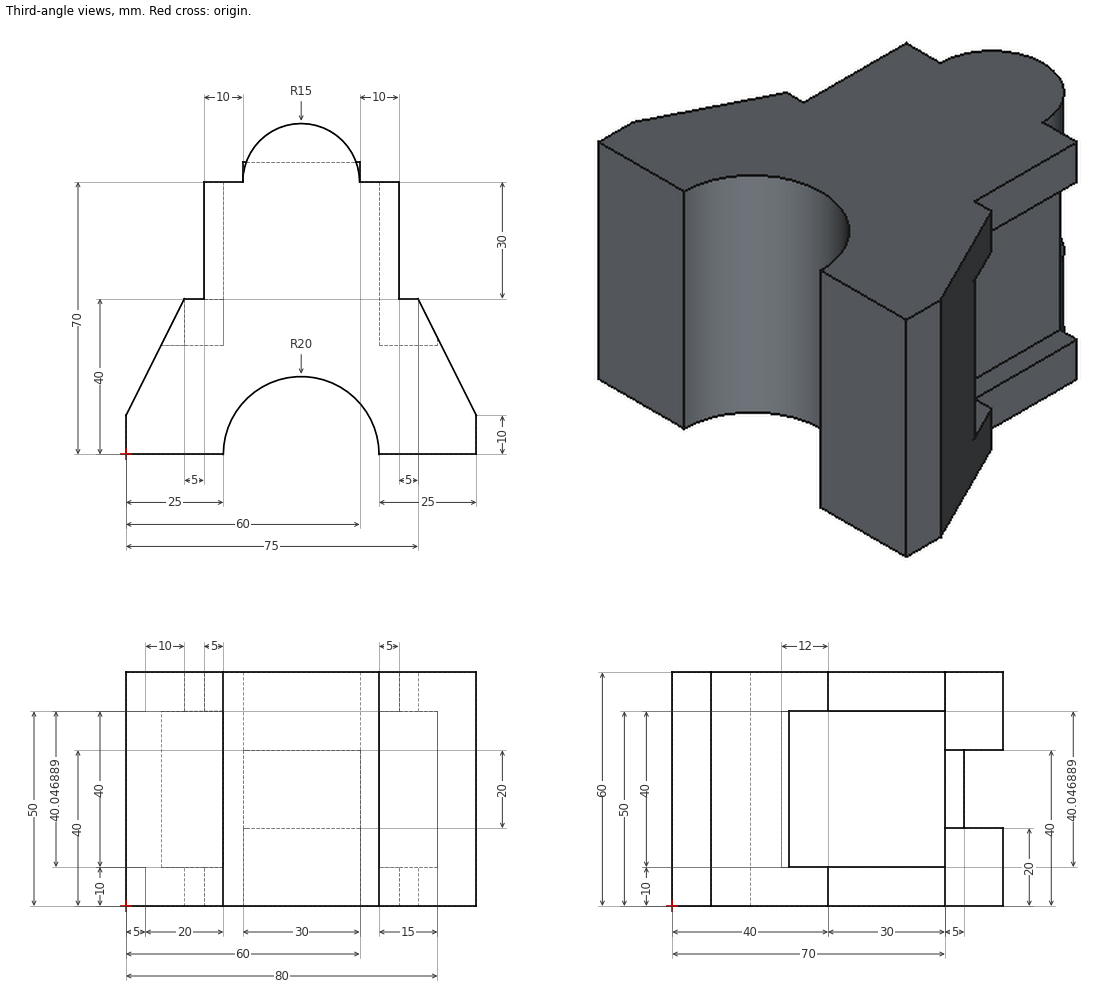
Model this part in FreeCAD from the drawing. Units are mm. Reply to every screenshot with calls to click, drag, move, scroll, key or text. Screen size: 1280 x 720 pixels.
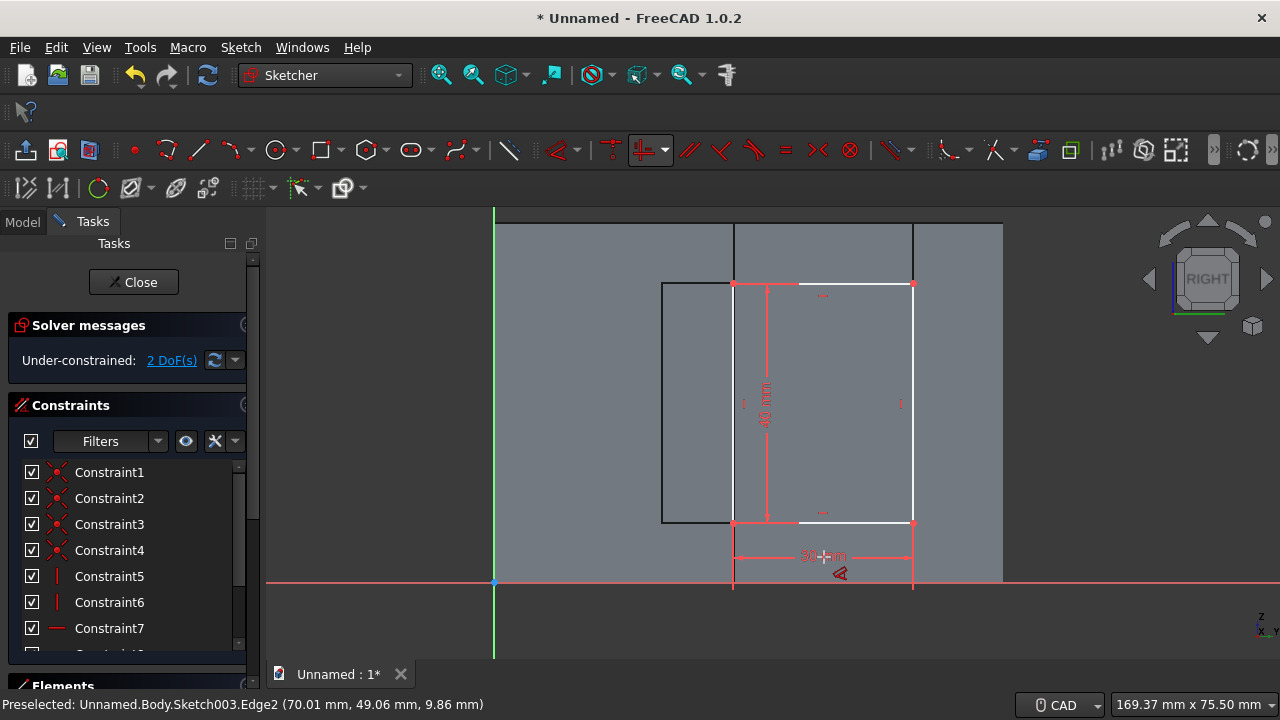
click(733, 284)
click(614, 617)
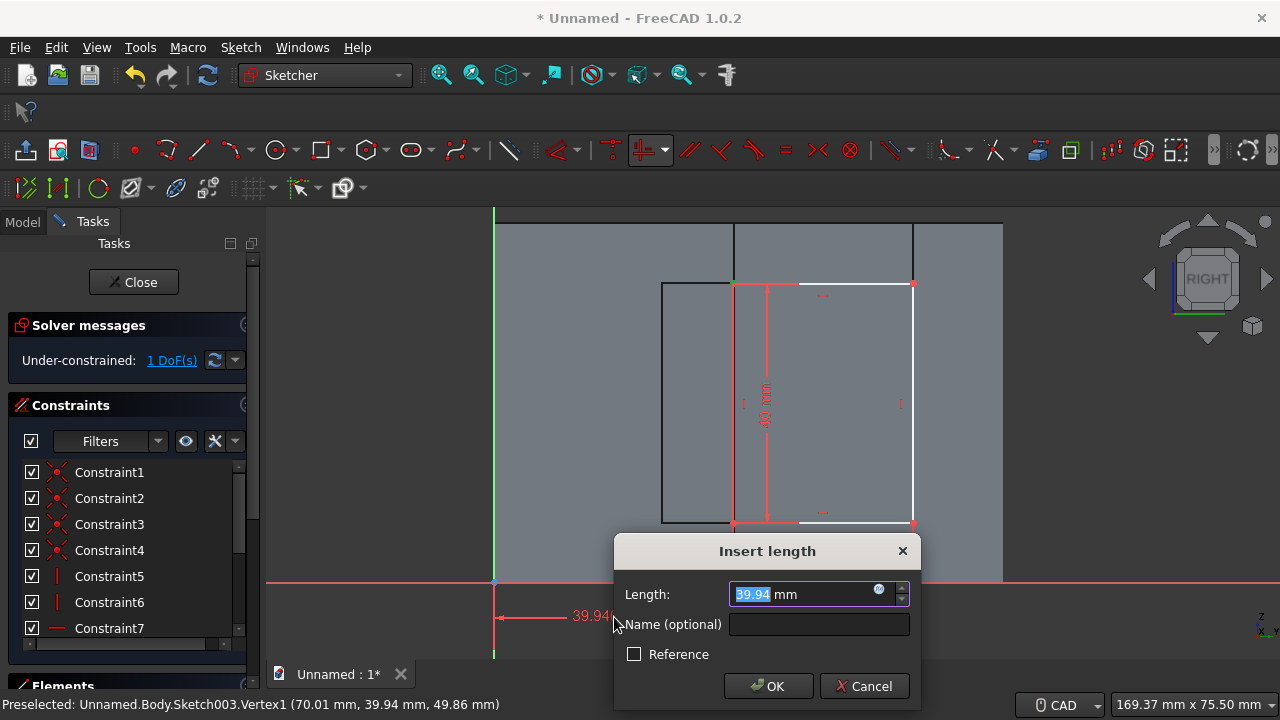
text(40)
key(Return)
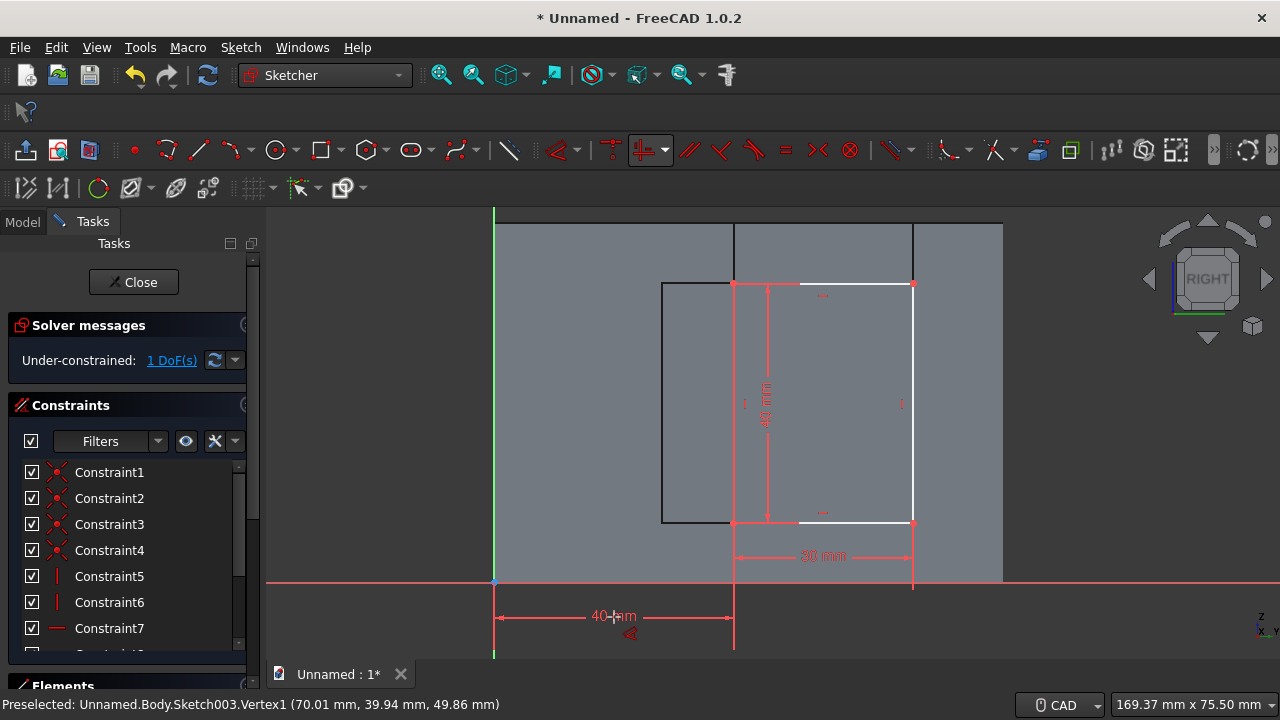
click(734, 284)
click(460, 433)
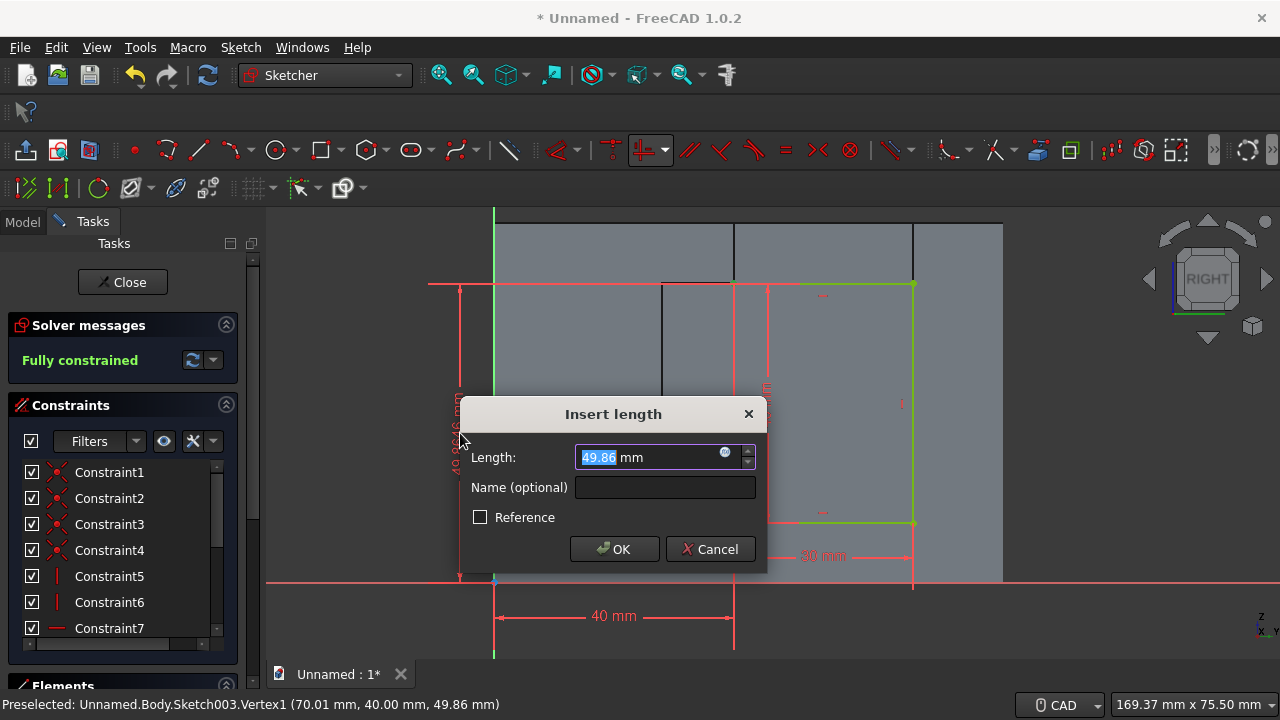
text(50)
key(Return)
key(Escape)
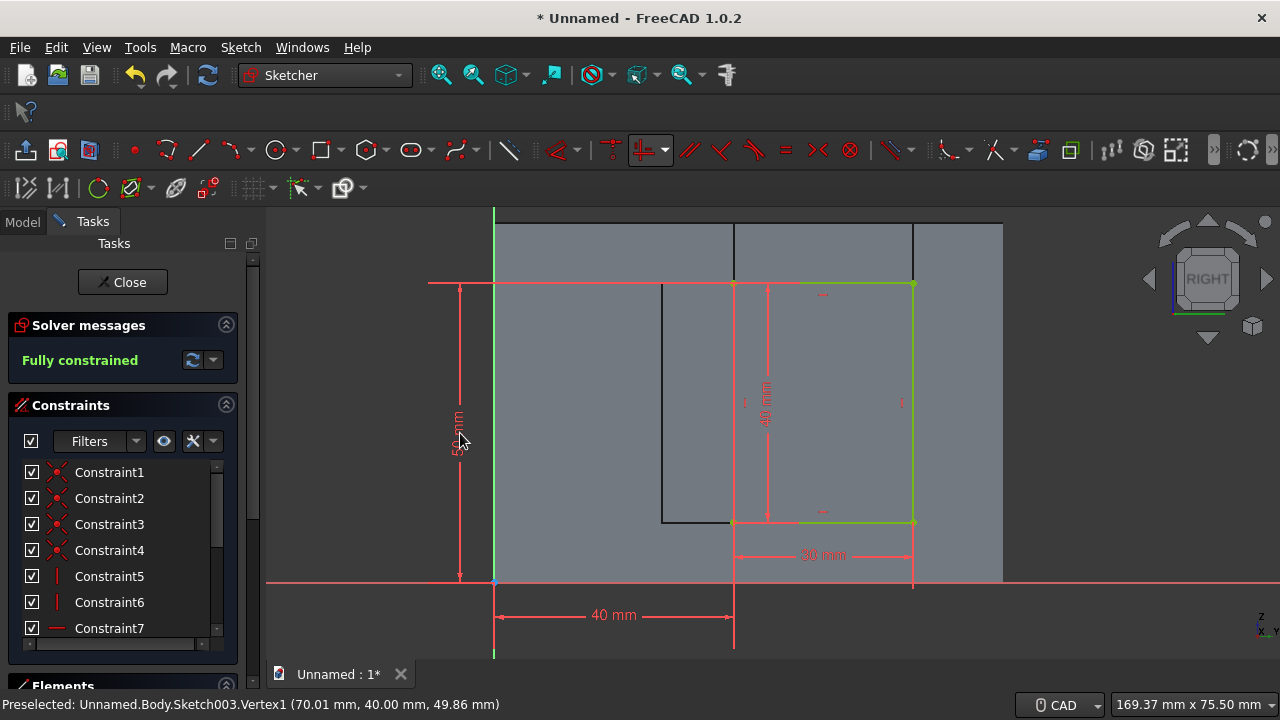
click(123, 282)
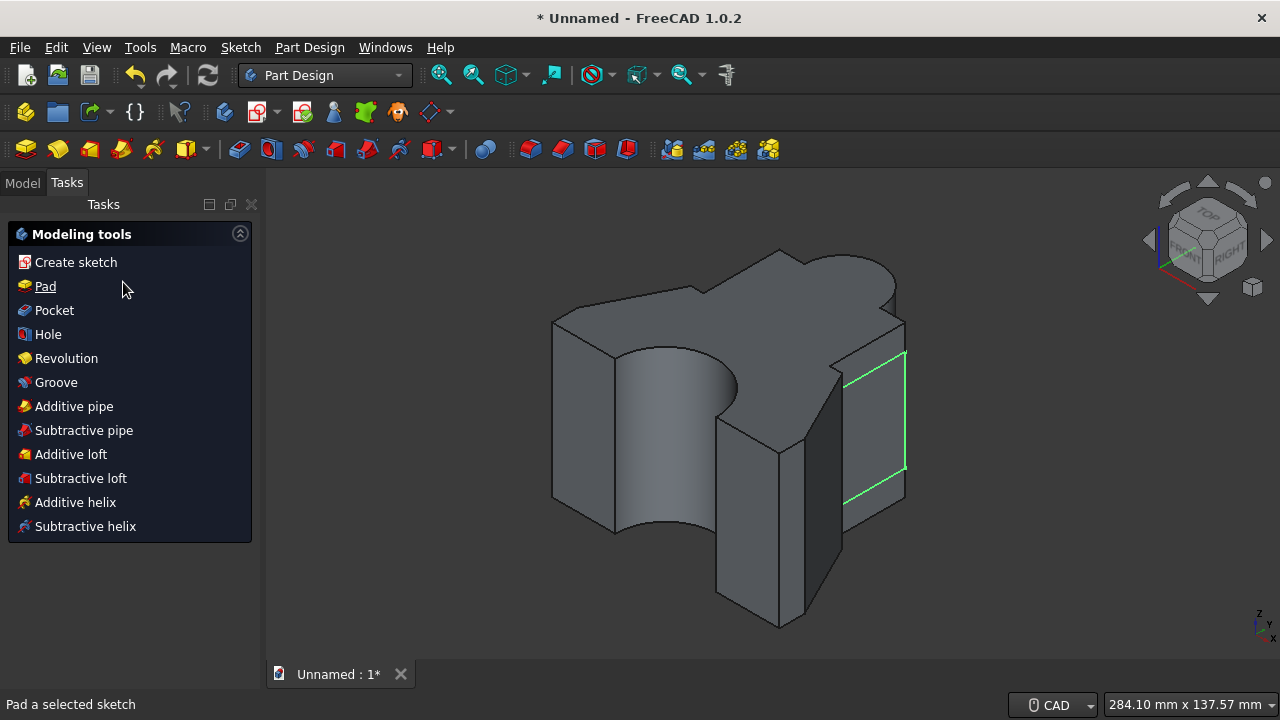
click(240, 150)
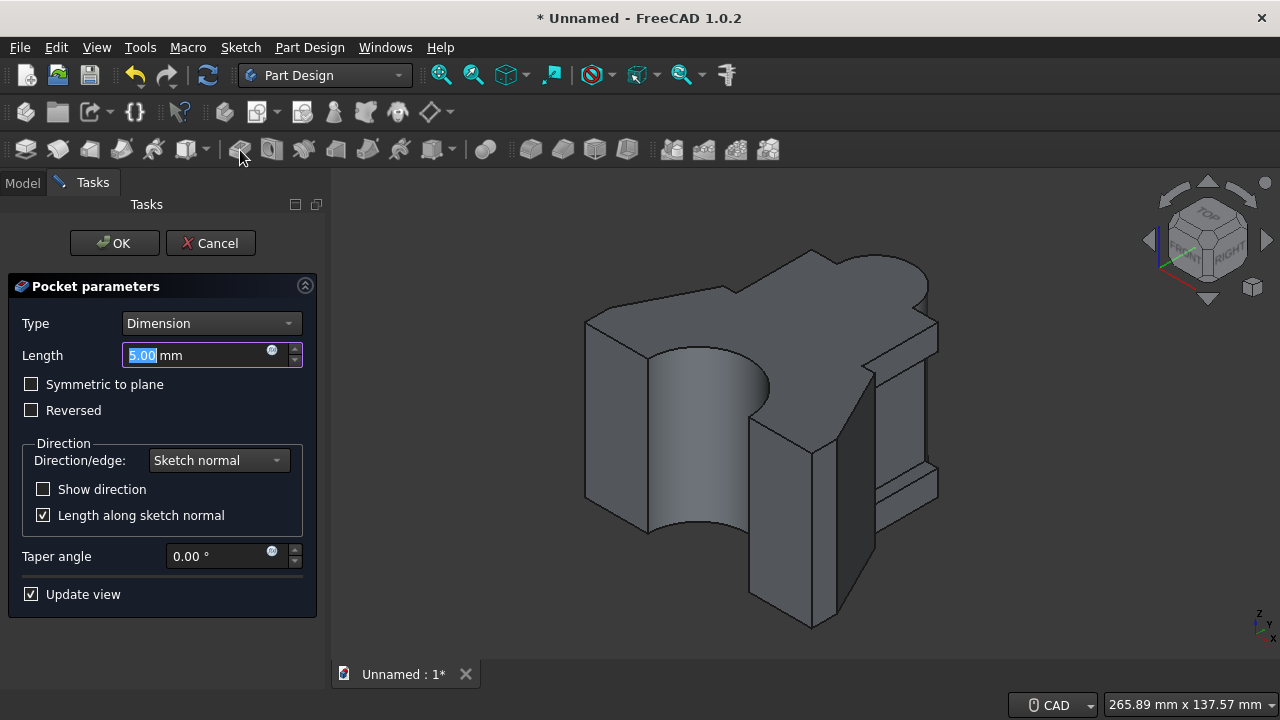
text(5)
key(Tab)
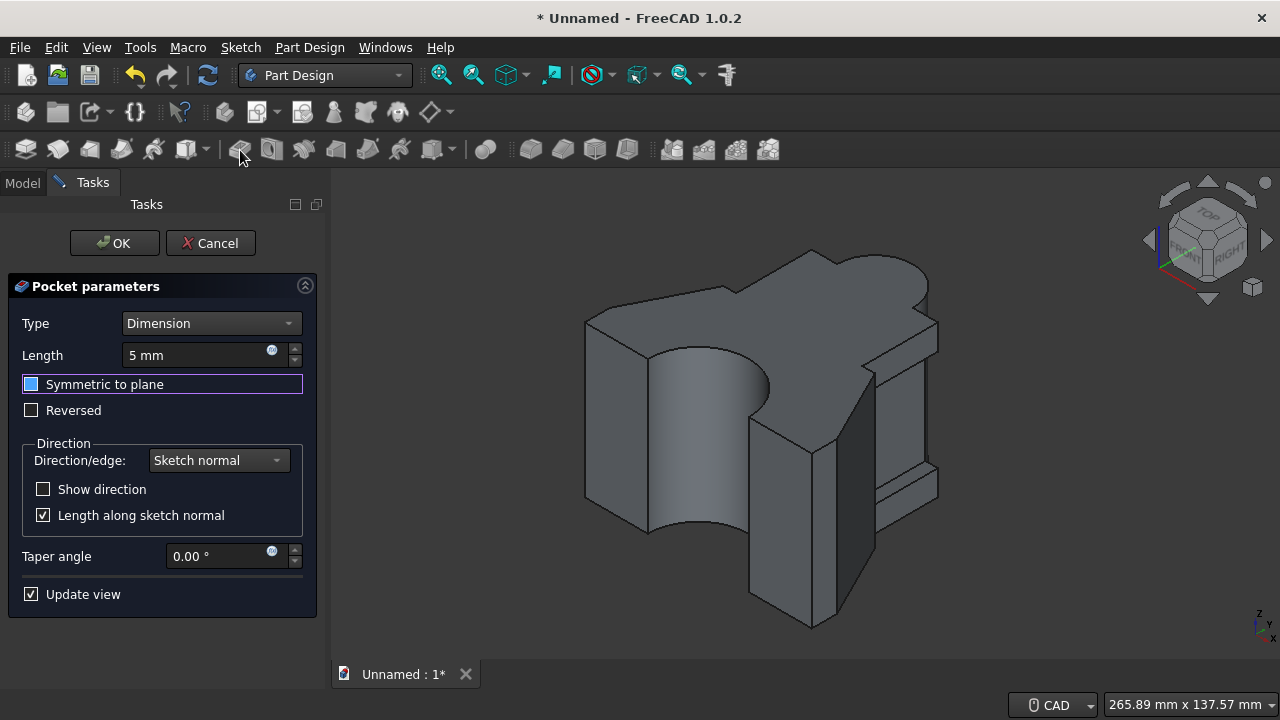
click(115, 243)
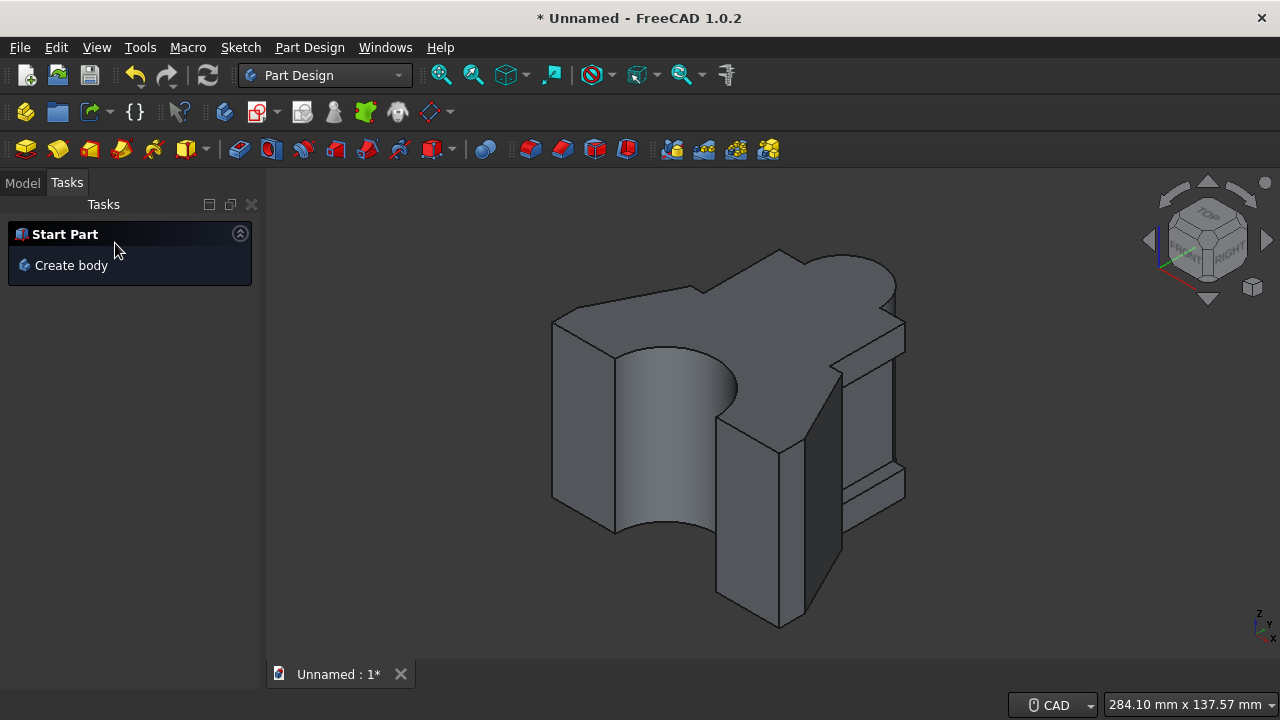
key(4)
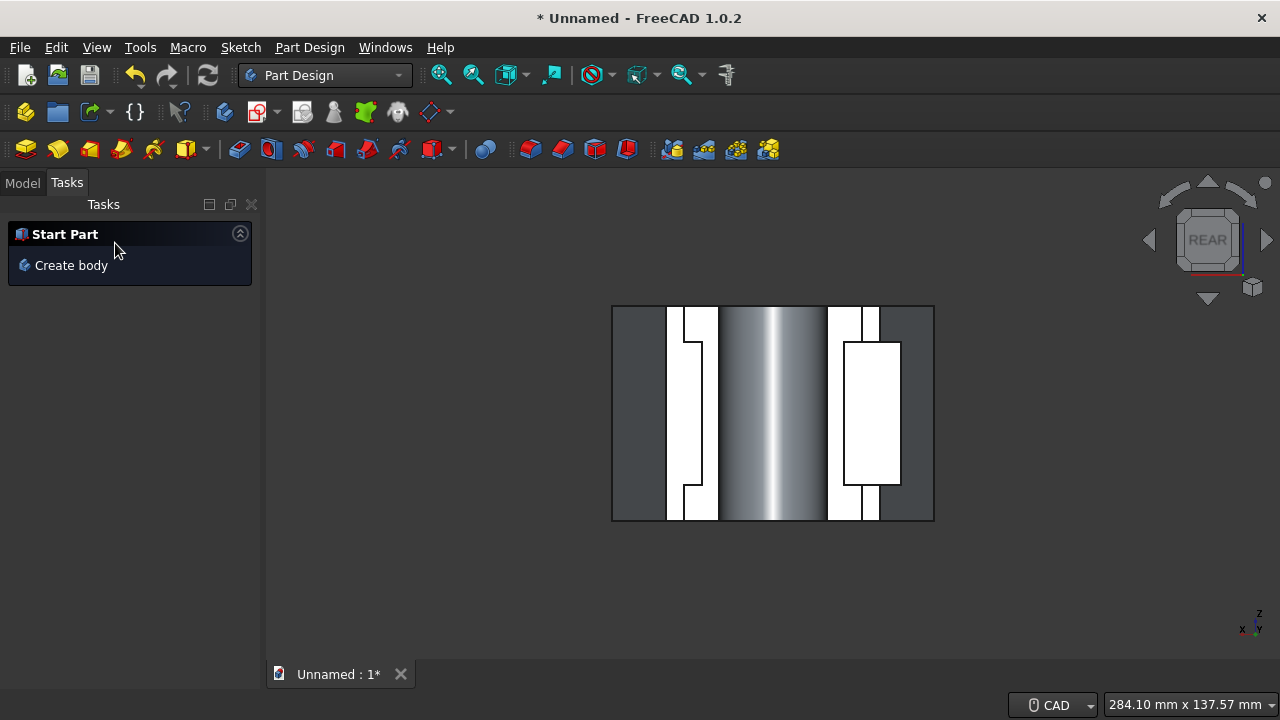
key(v)
key(f)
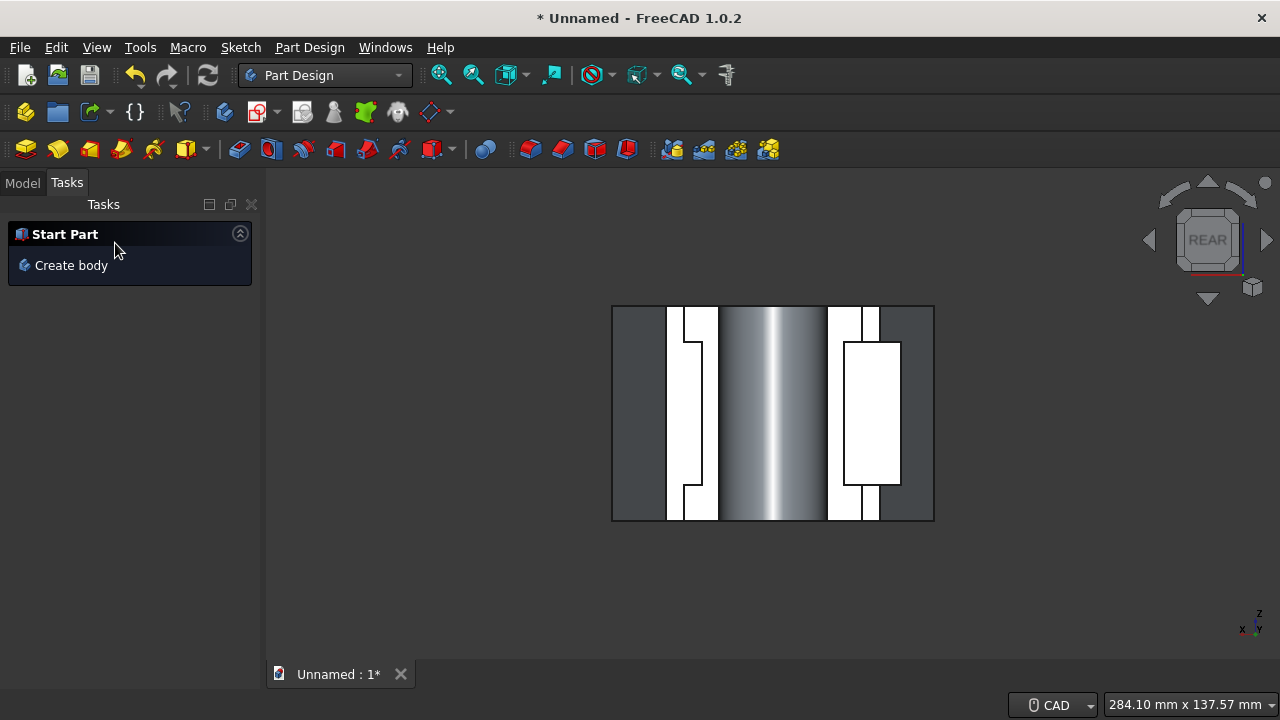
click(684, 382)